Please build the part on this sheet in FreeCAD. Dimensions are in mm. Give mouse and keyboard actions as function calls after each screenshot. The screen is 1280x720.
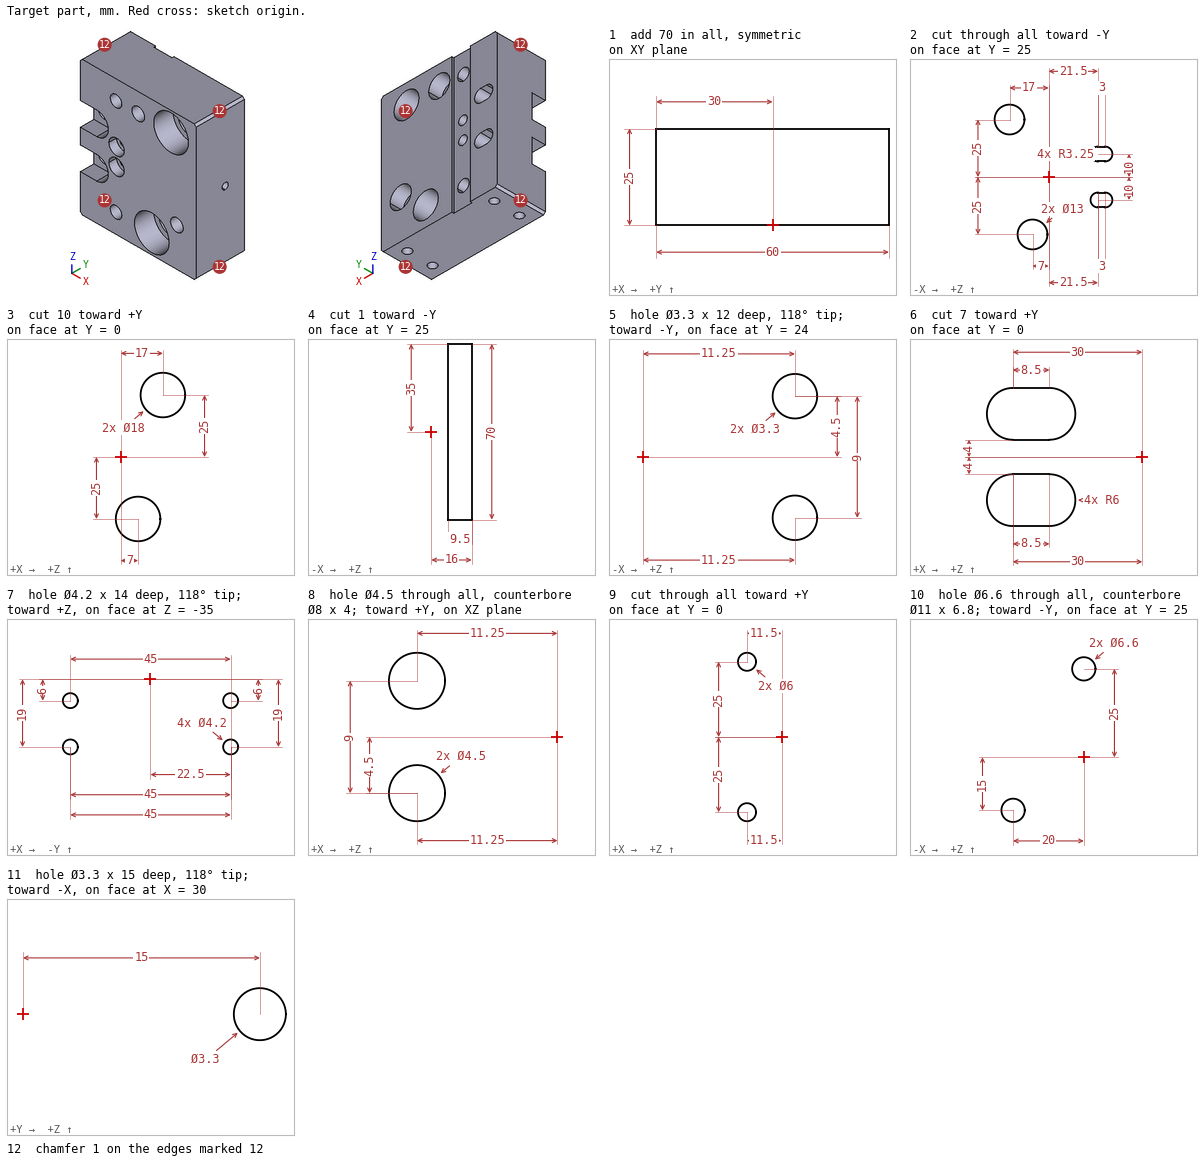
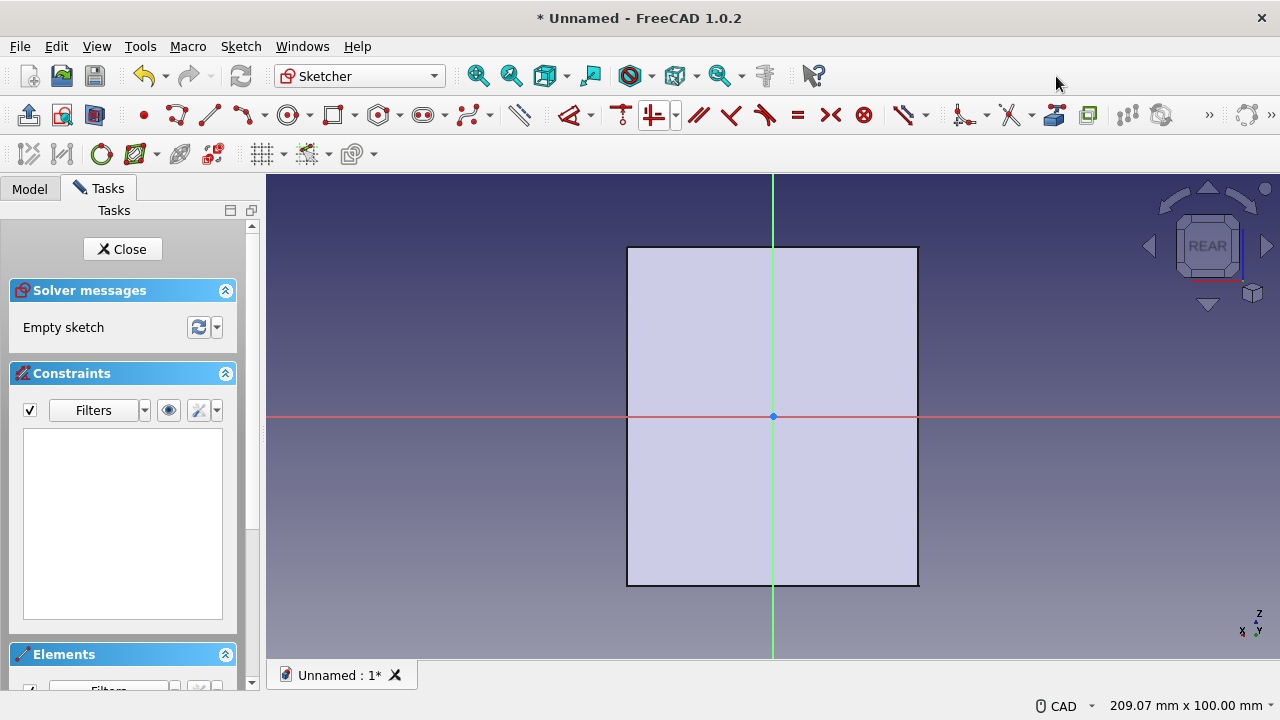
key(g)
key(s)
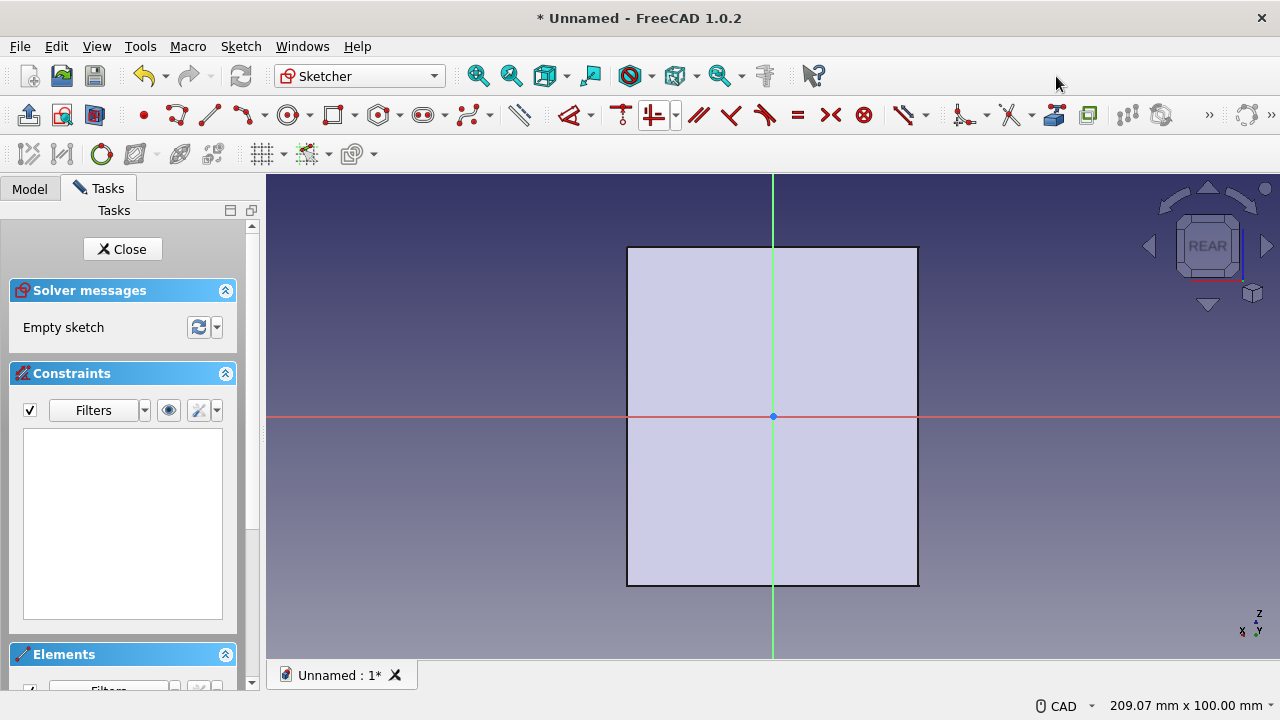
scroll(877, 465, up, 2)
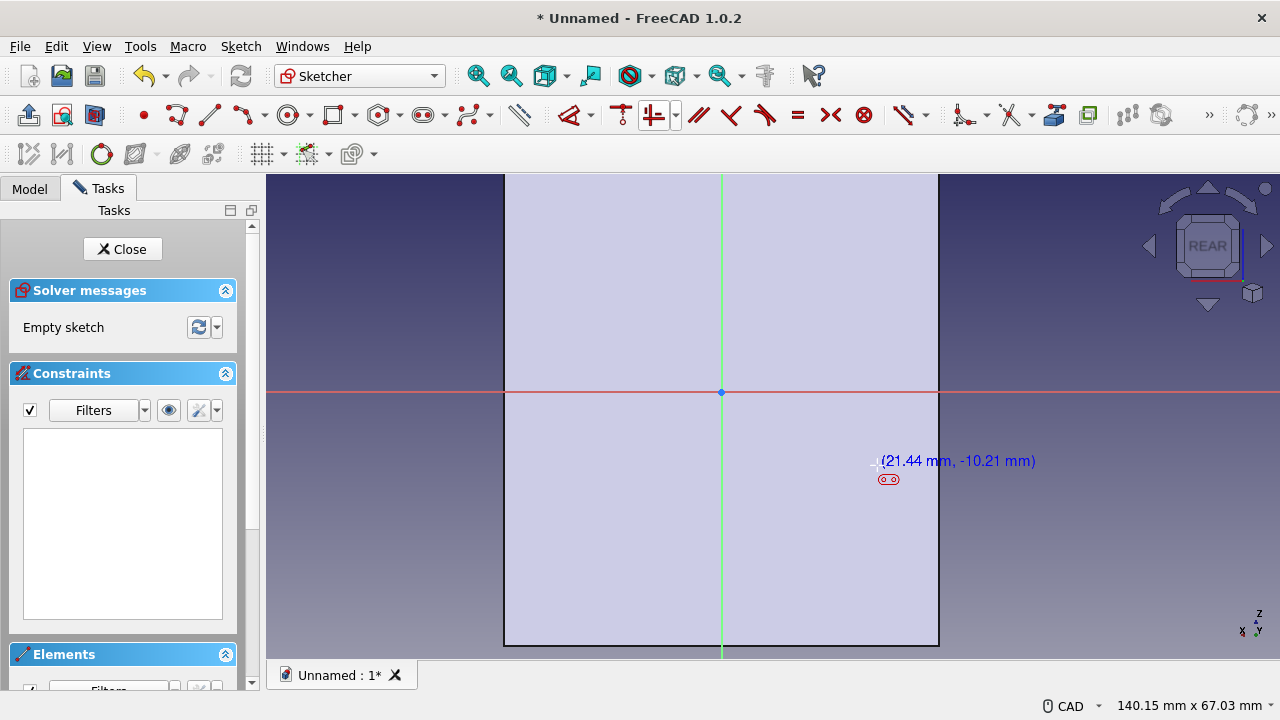
click(877, 465)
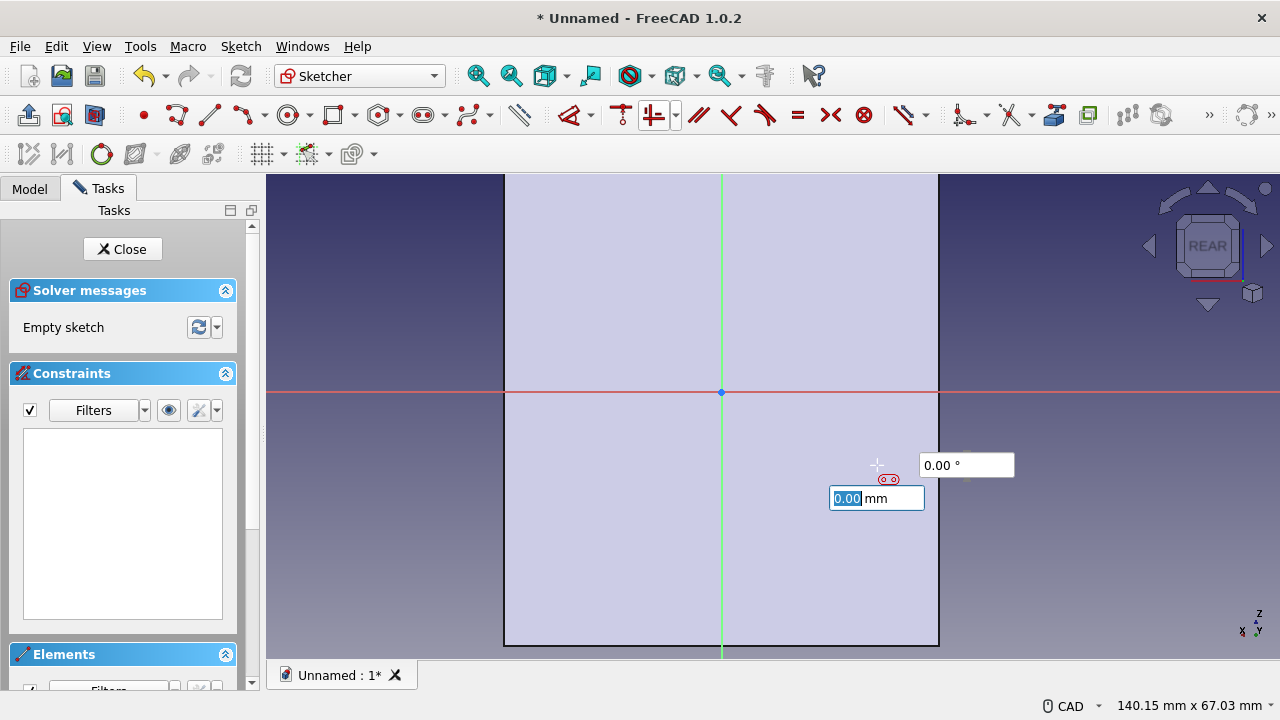
click(899, 465)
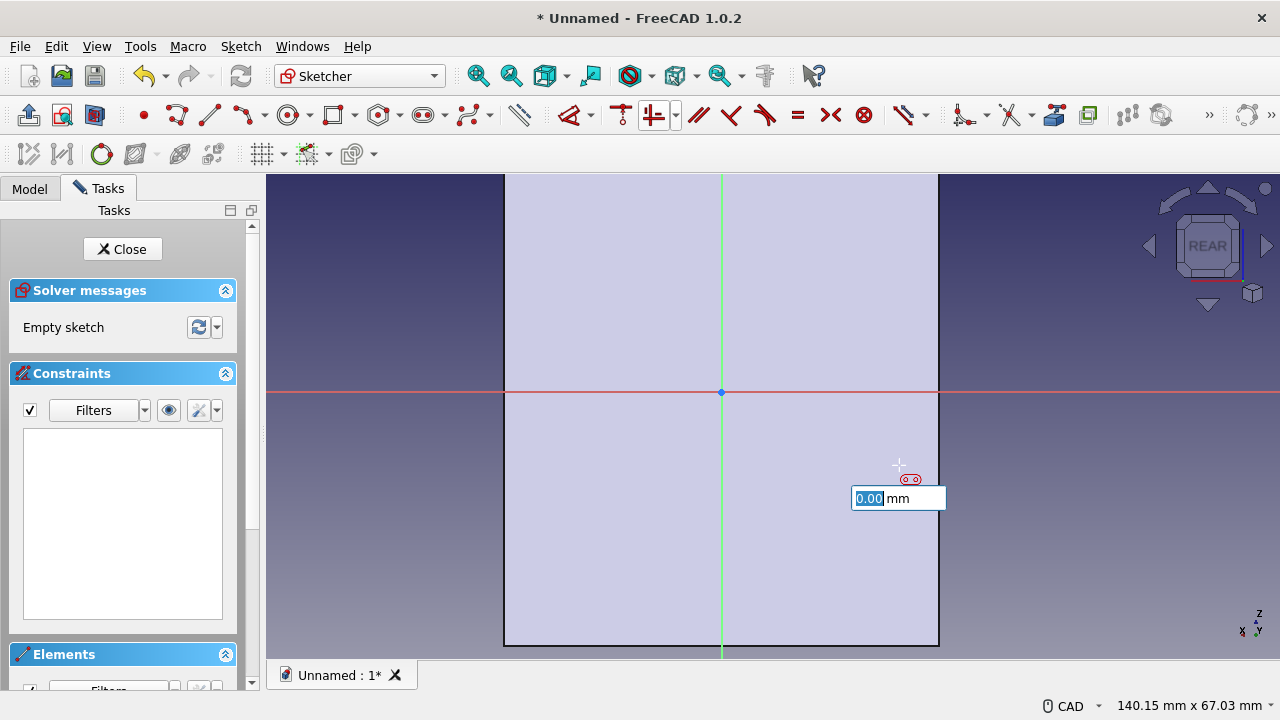
click(888, 488)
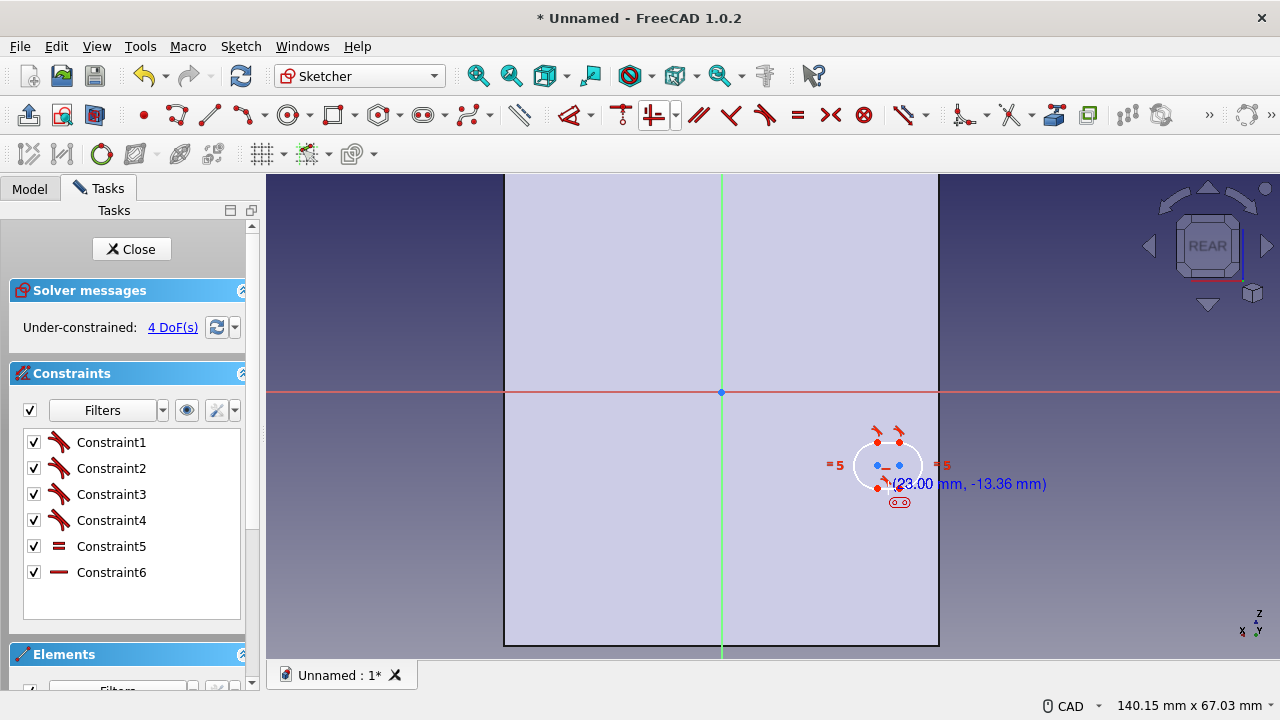
click(877, 320)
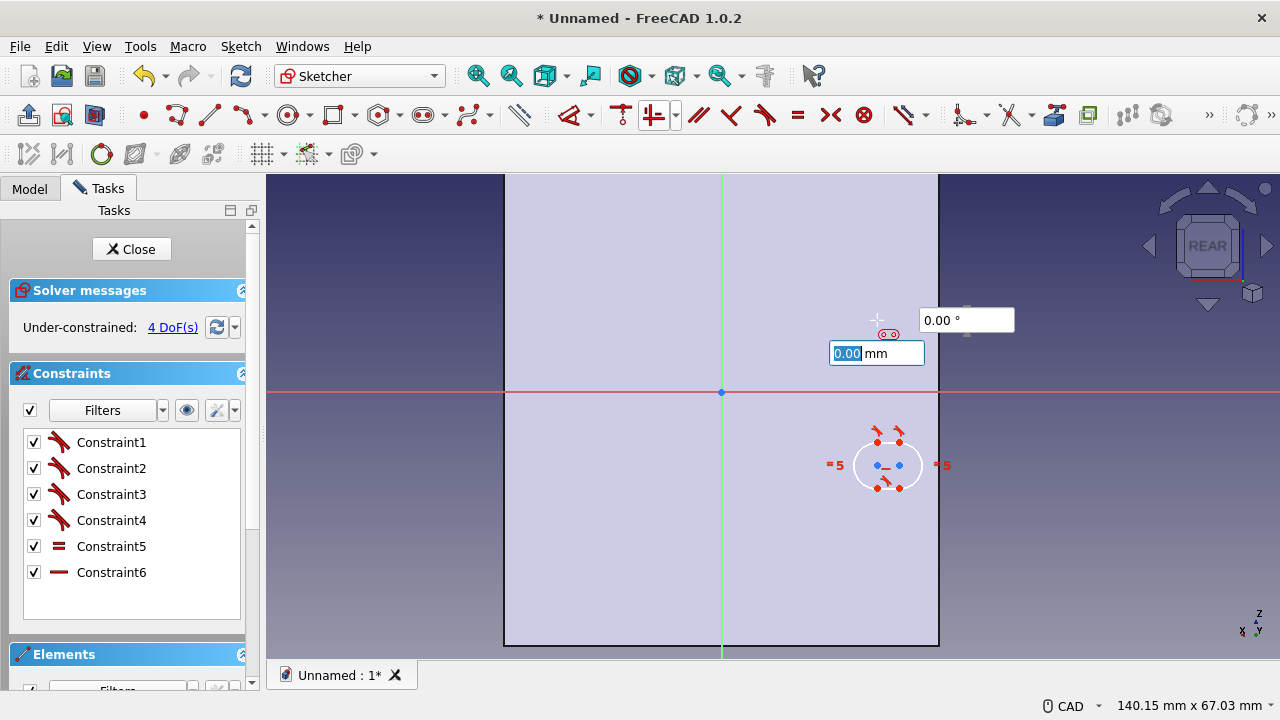
click(899, 320)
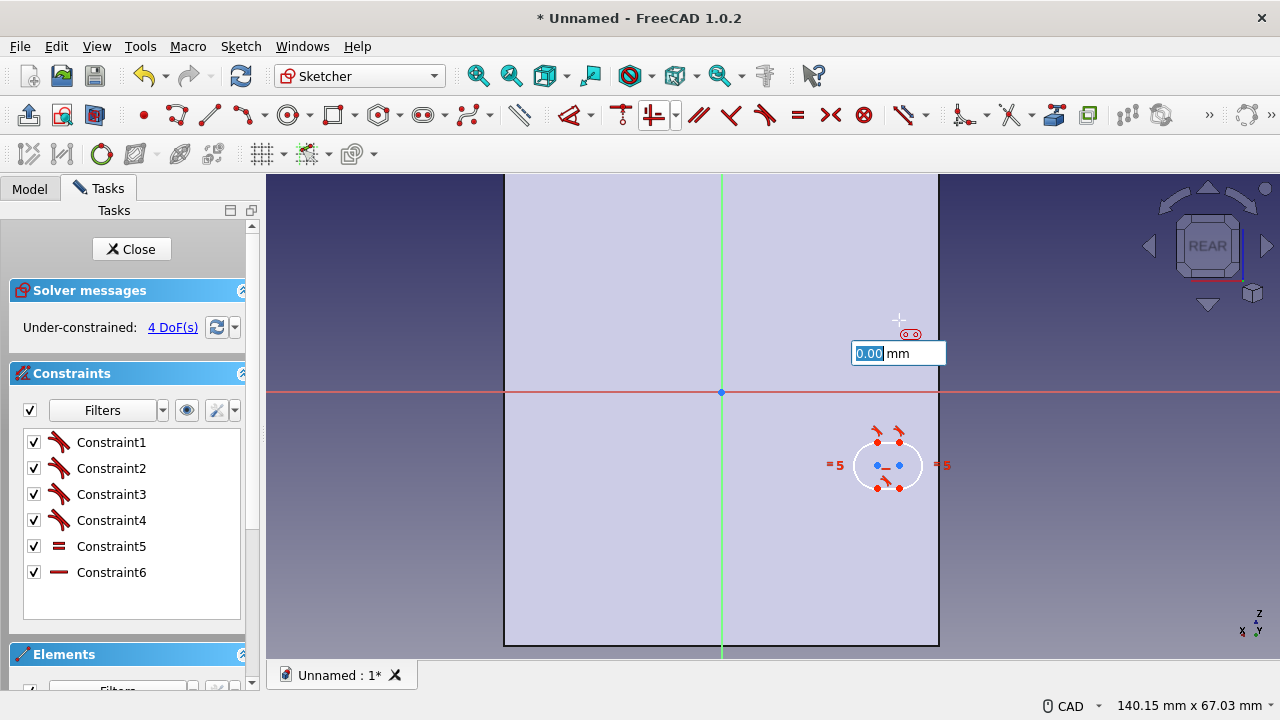
click(888, 344)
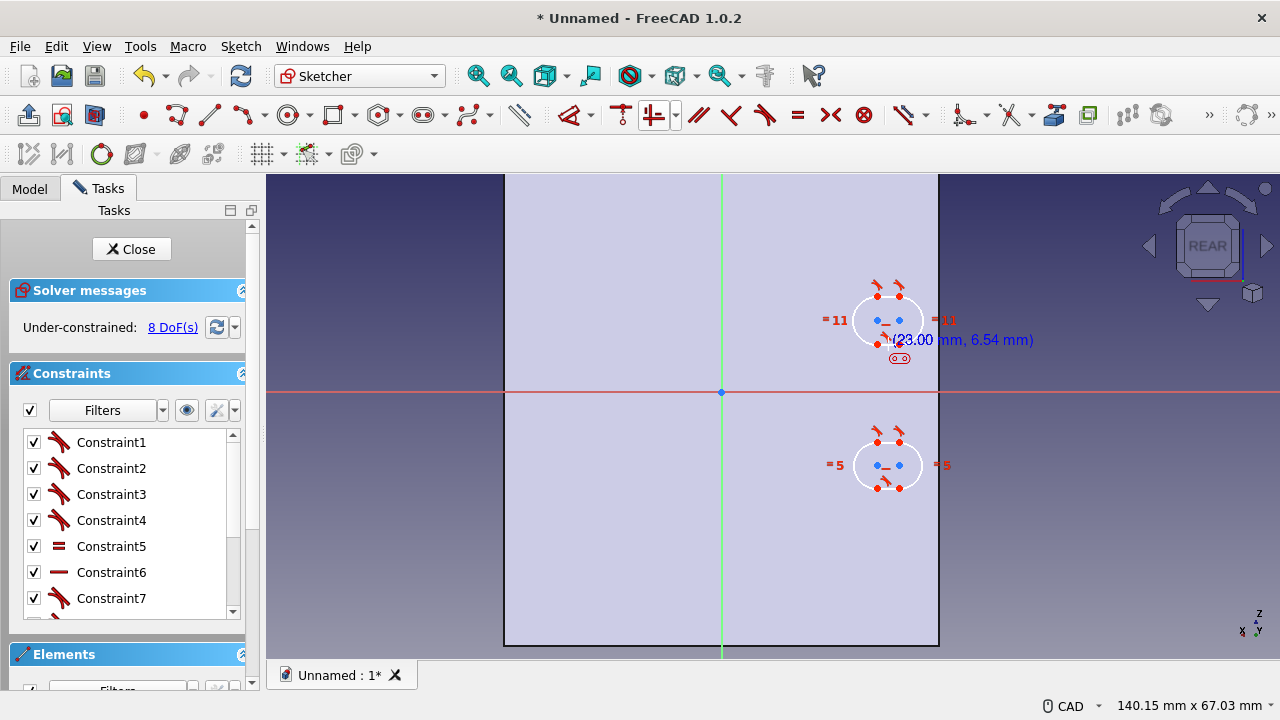
key(g)
key(c)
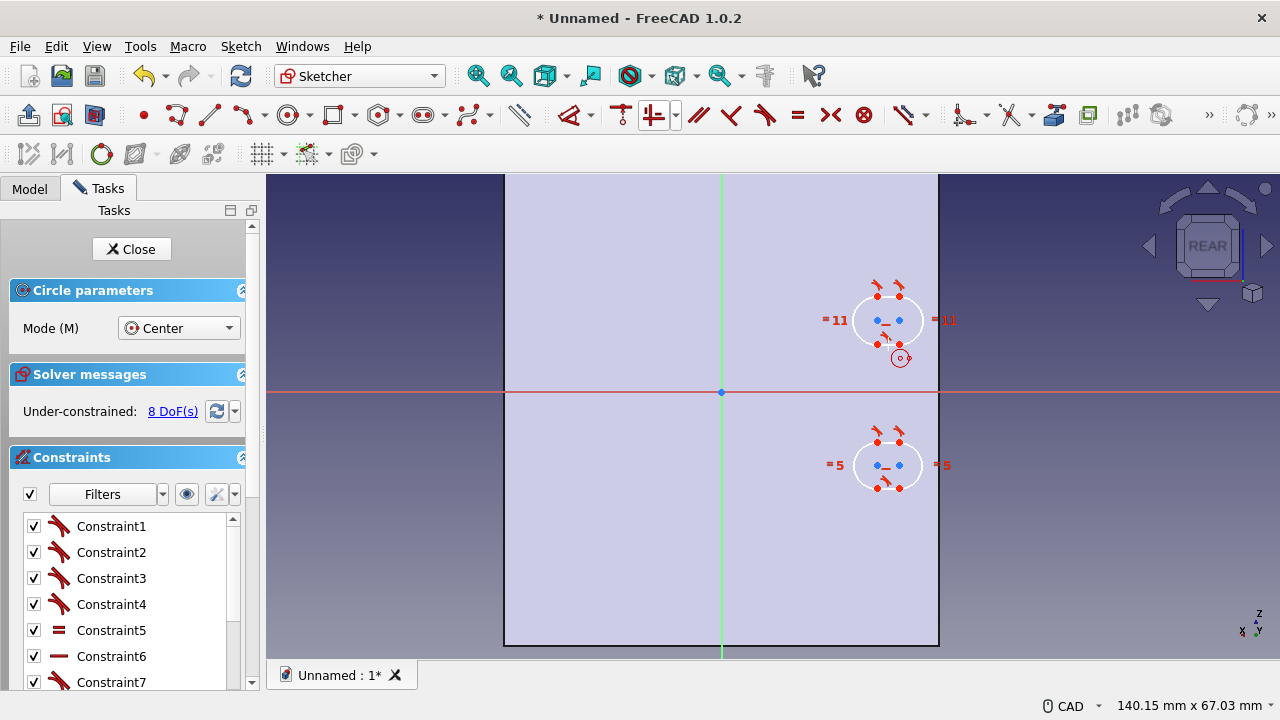
click(671, 573)
move(704, 540)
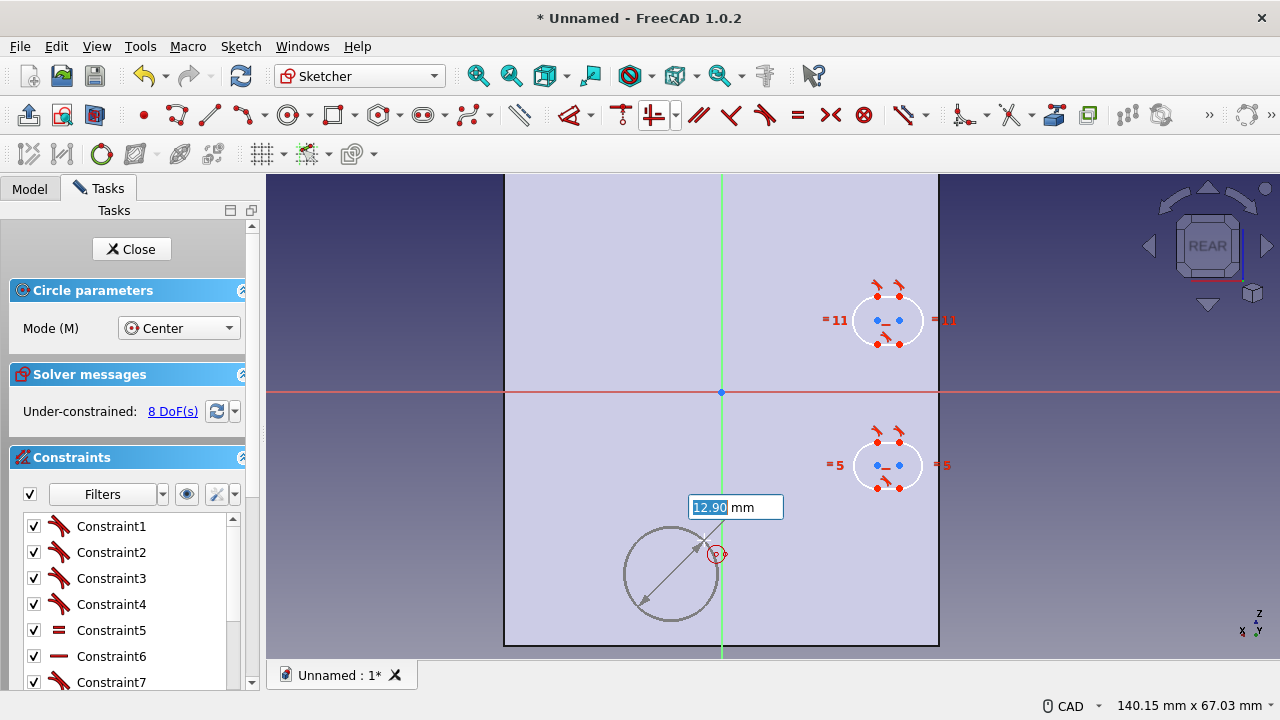
text(13)
key(Return)